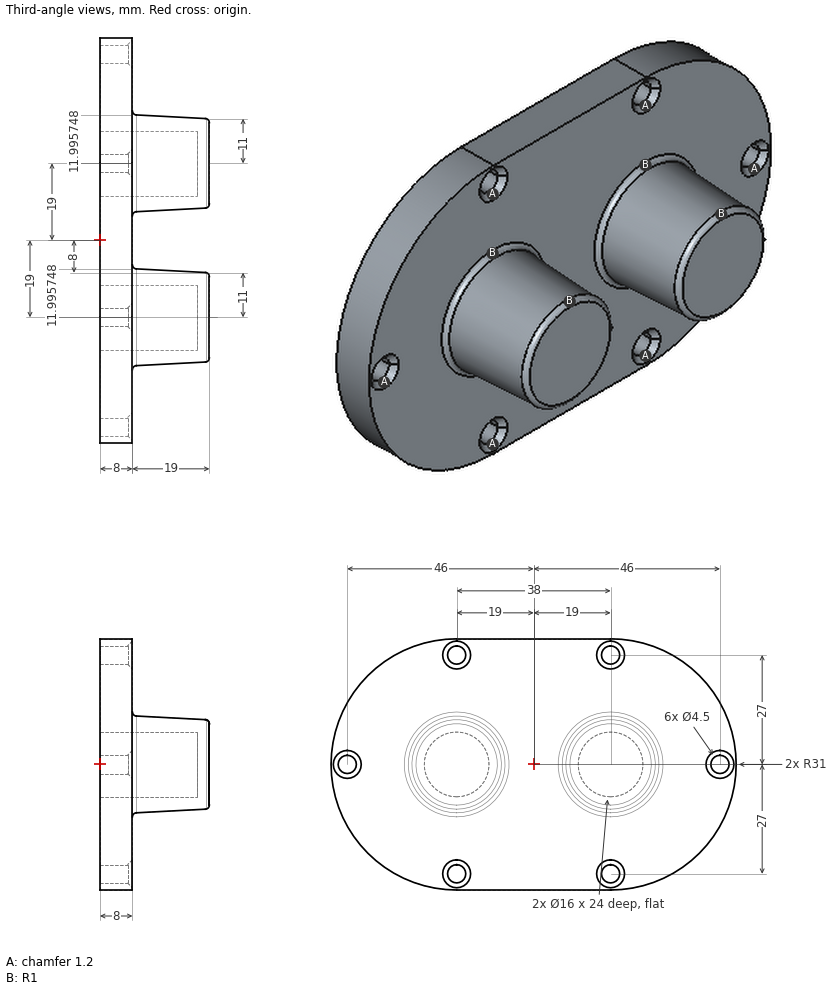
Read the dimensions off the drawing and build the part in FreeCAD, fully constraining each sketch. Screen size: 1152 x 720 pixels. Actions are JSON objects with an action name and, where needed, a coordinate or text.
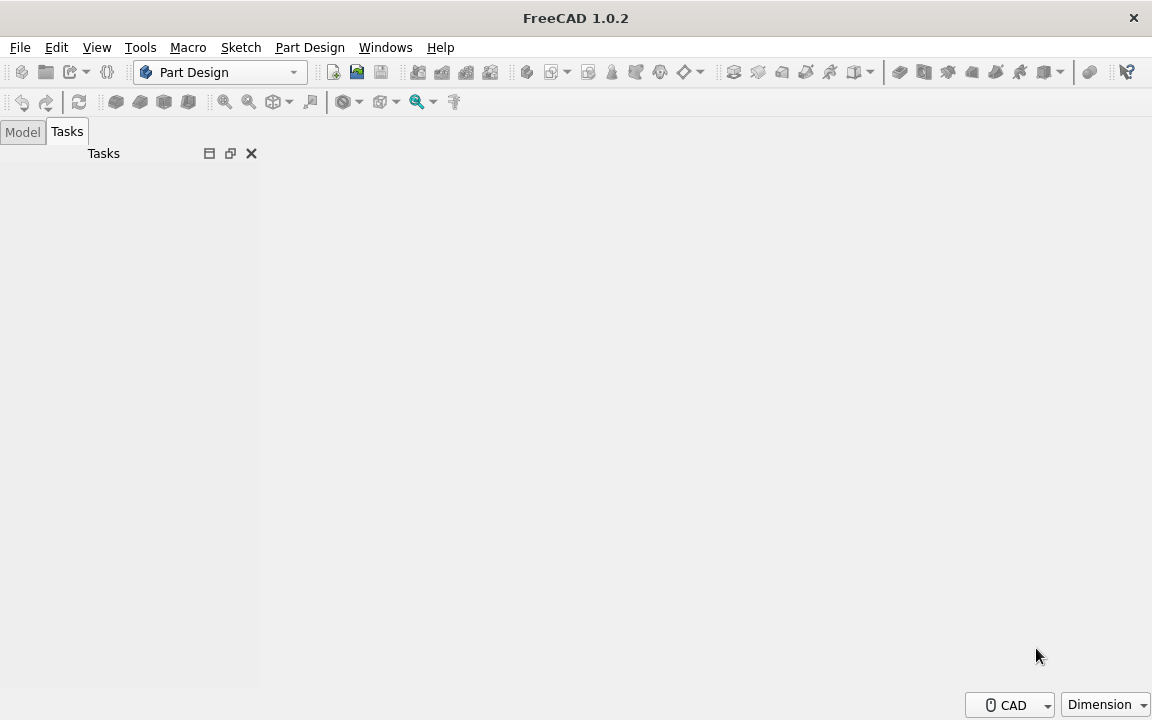
{"action": "left_click", "coordinate": [334, 72]}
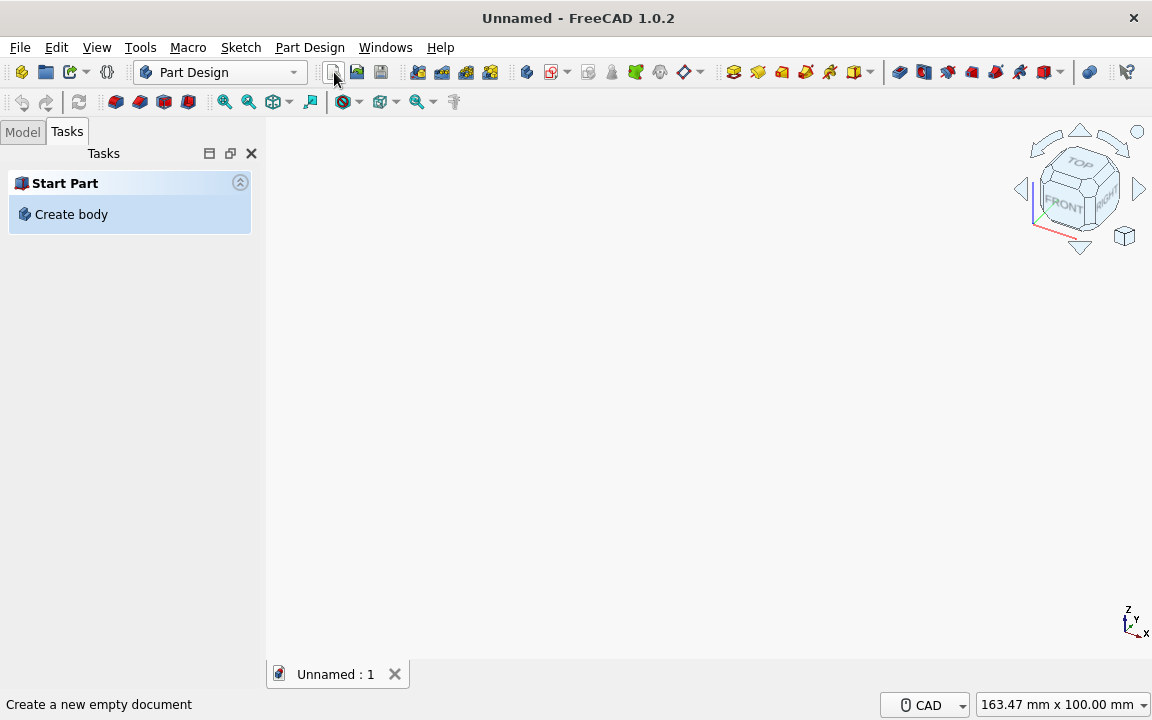
{"action": "left_click", "coordinate": [528, 72]}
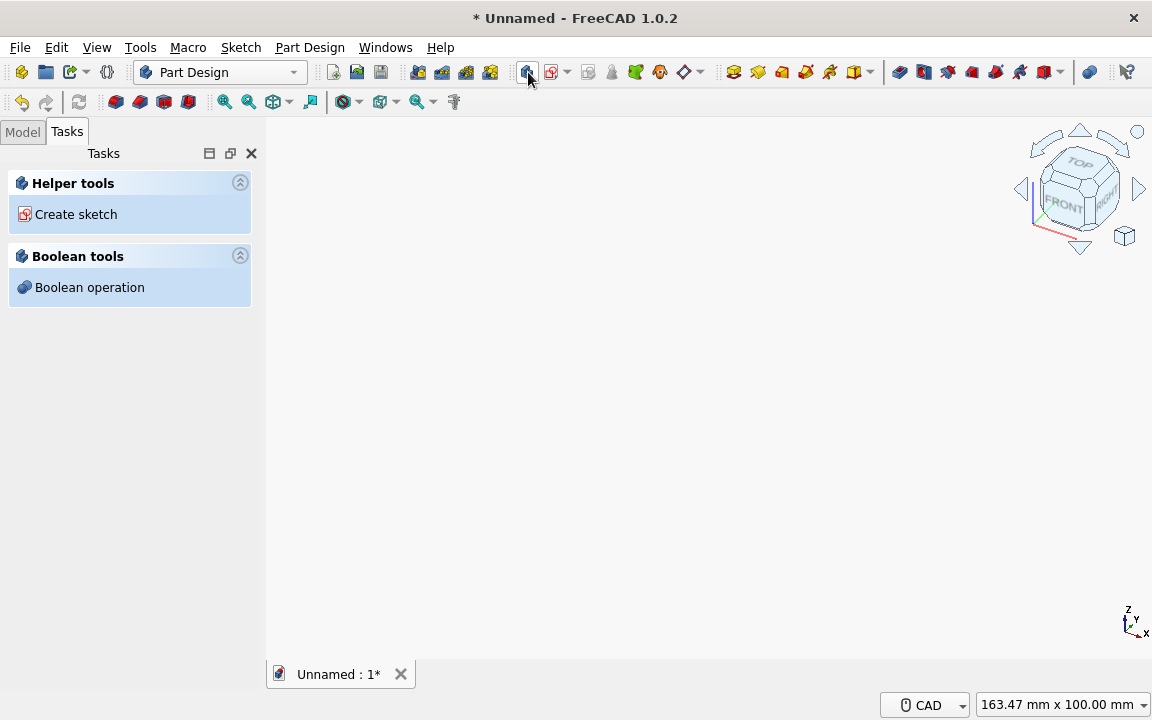
{"action": "left_click", "coordinate": [23, 131]}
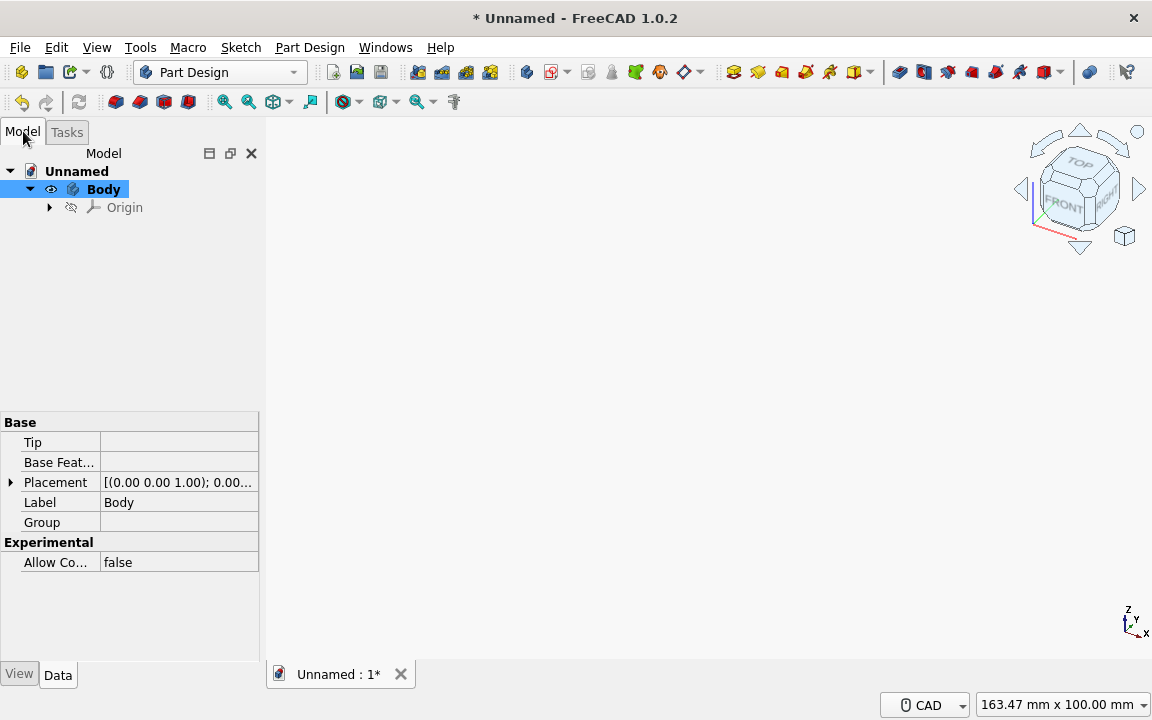
{"action": "left_click", "coordinate": [50, 207]}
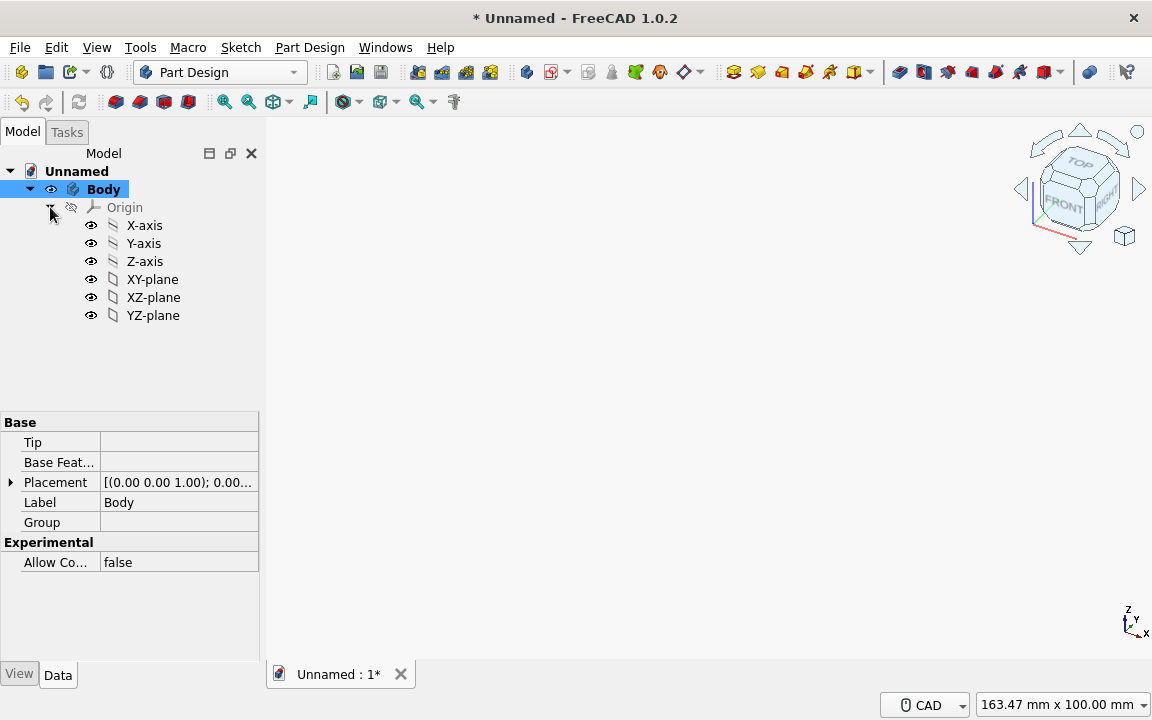
{"action": "left_click", "coordinate": [136, 315]}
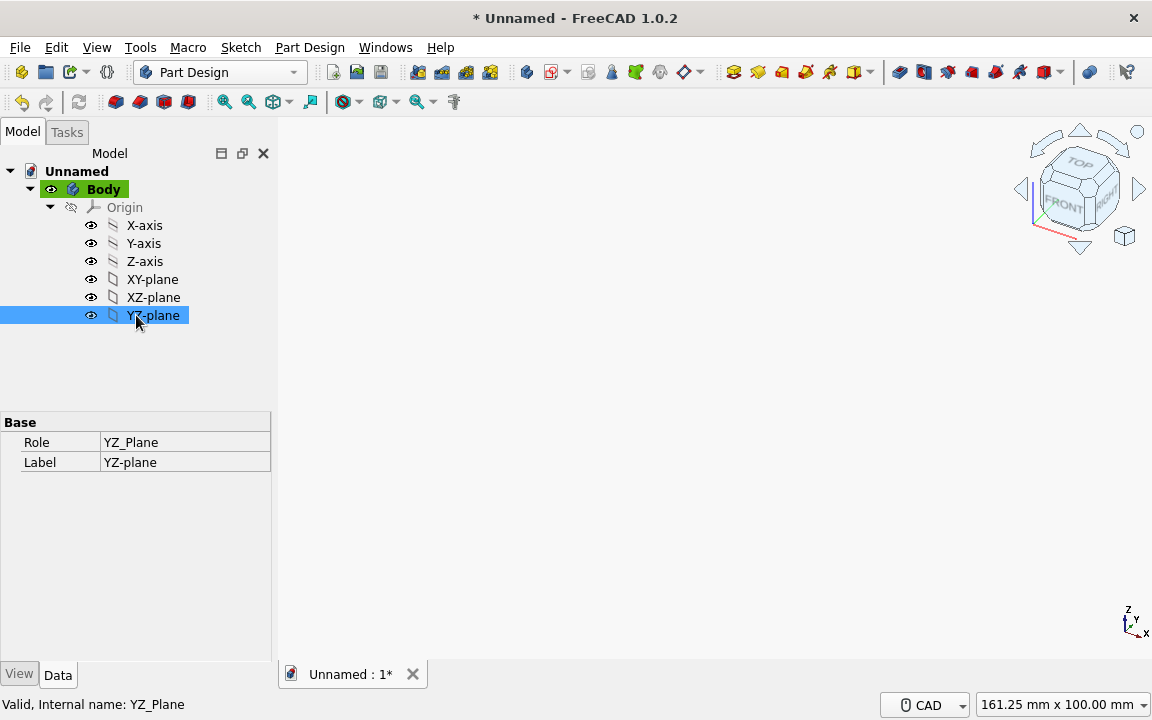
{"action": "left_click", "coordinate": [684, 72]}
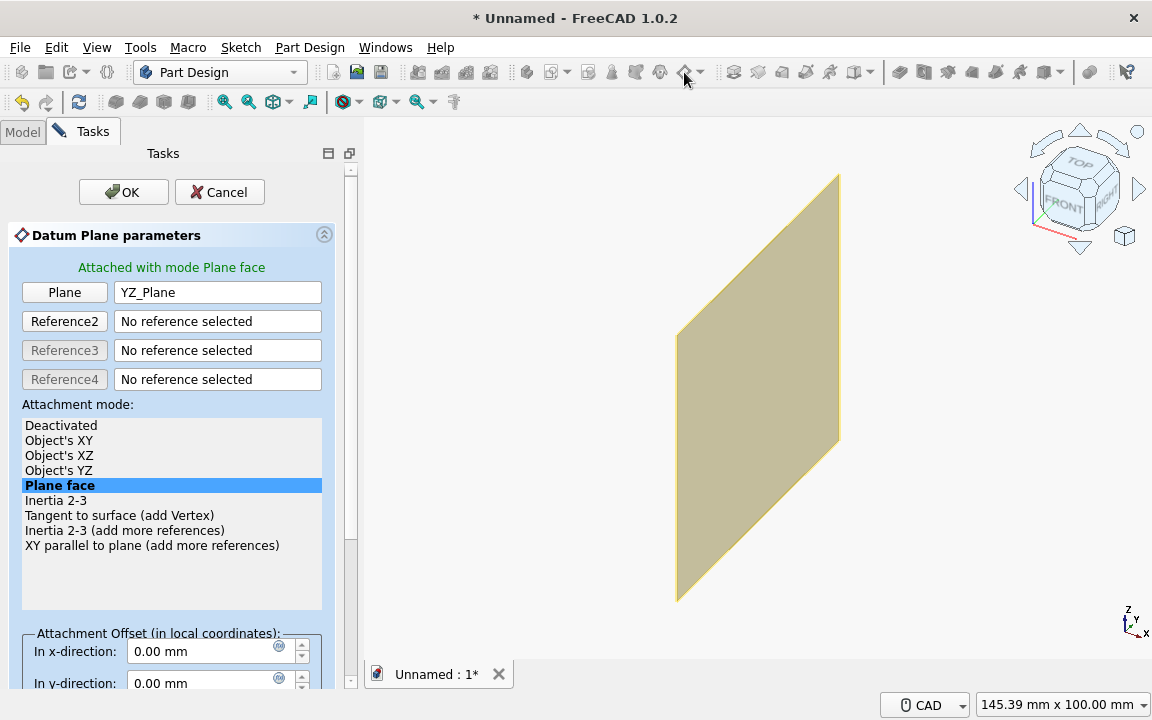
{"action": "scroll", "coordinate": [351, 426], "scroll_direction": "down", "scroll_amount": 2}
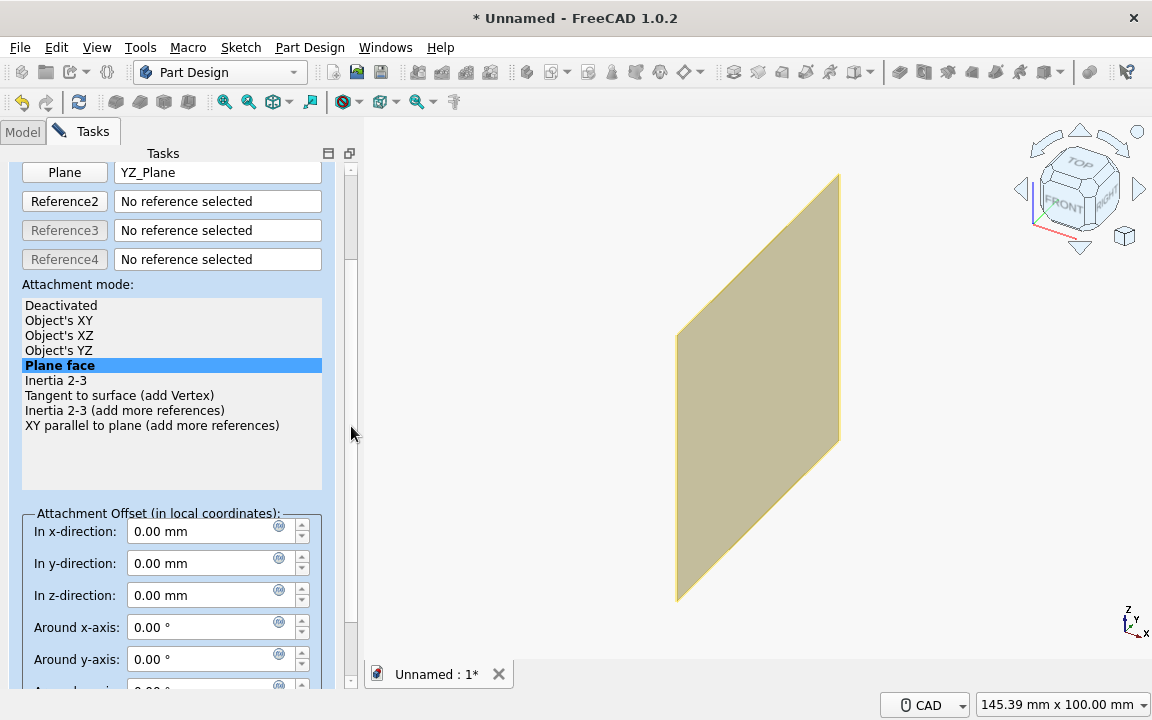
{"action": "triple_click", "coordinate": [210, 595]}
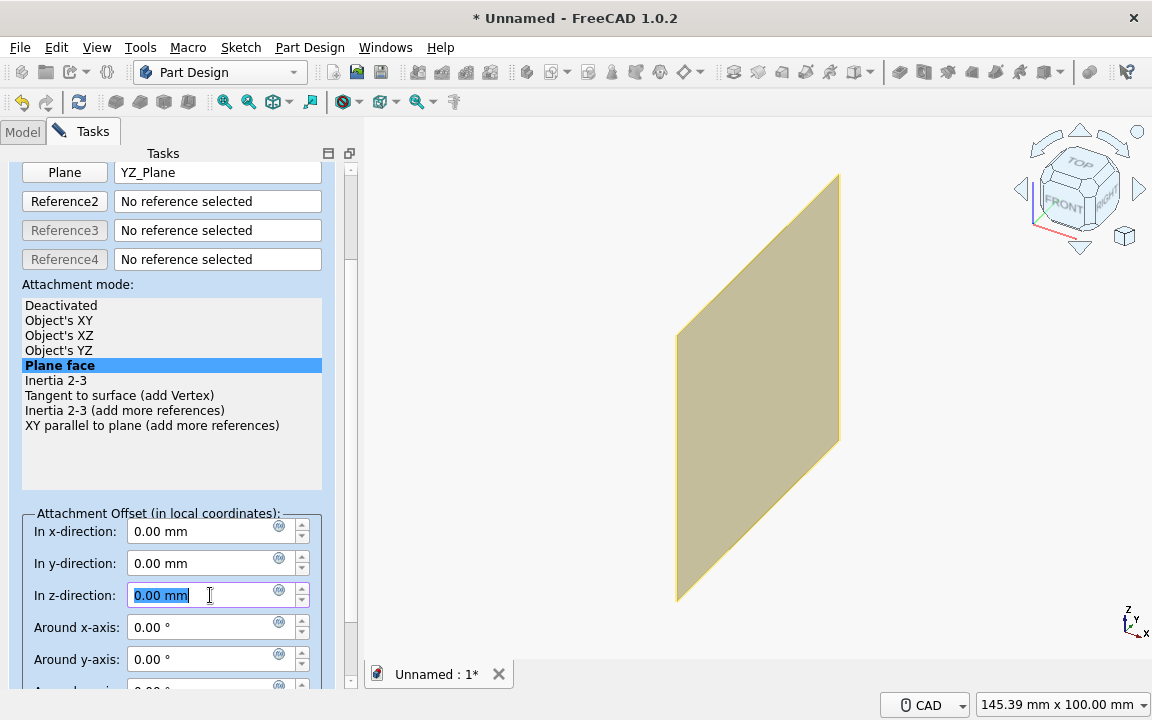
{"action": "type", "text": "8"}
{"action": "key", "text": "Tab"}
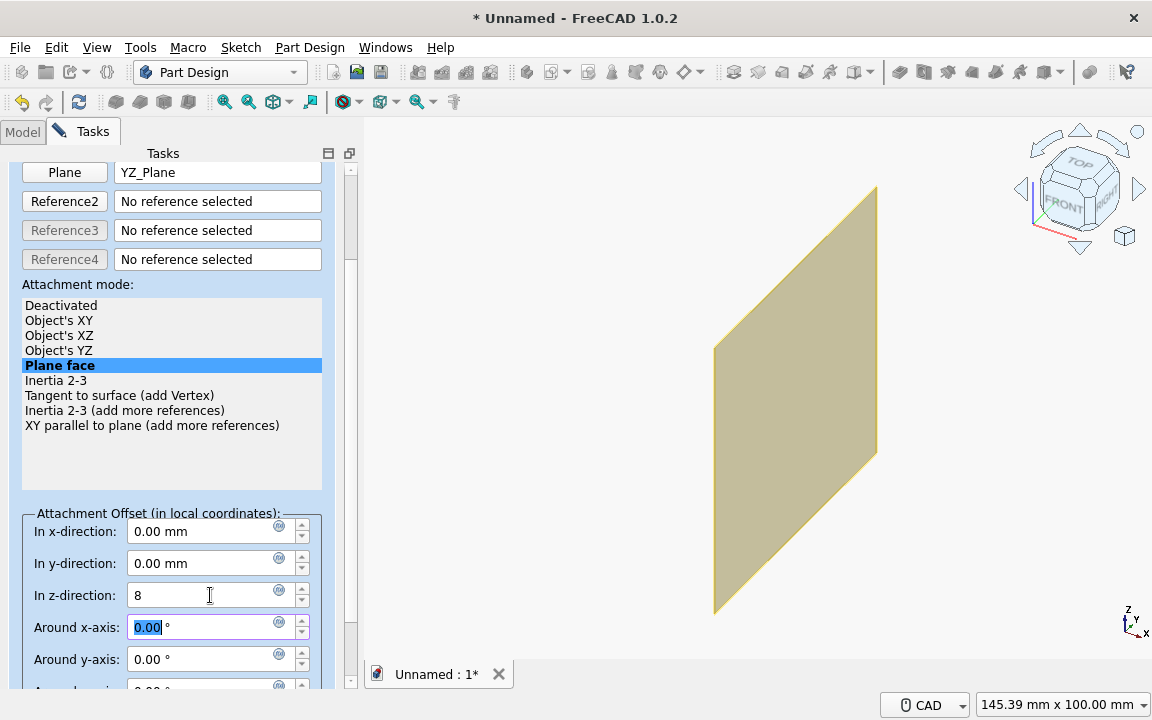
{"action": "scroll", "coordinate": [351, 426], "scroll_direction": "up", "scroll_amount": 3}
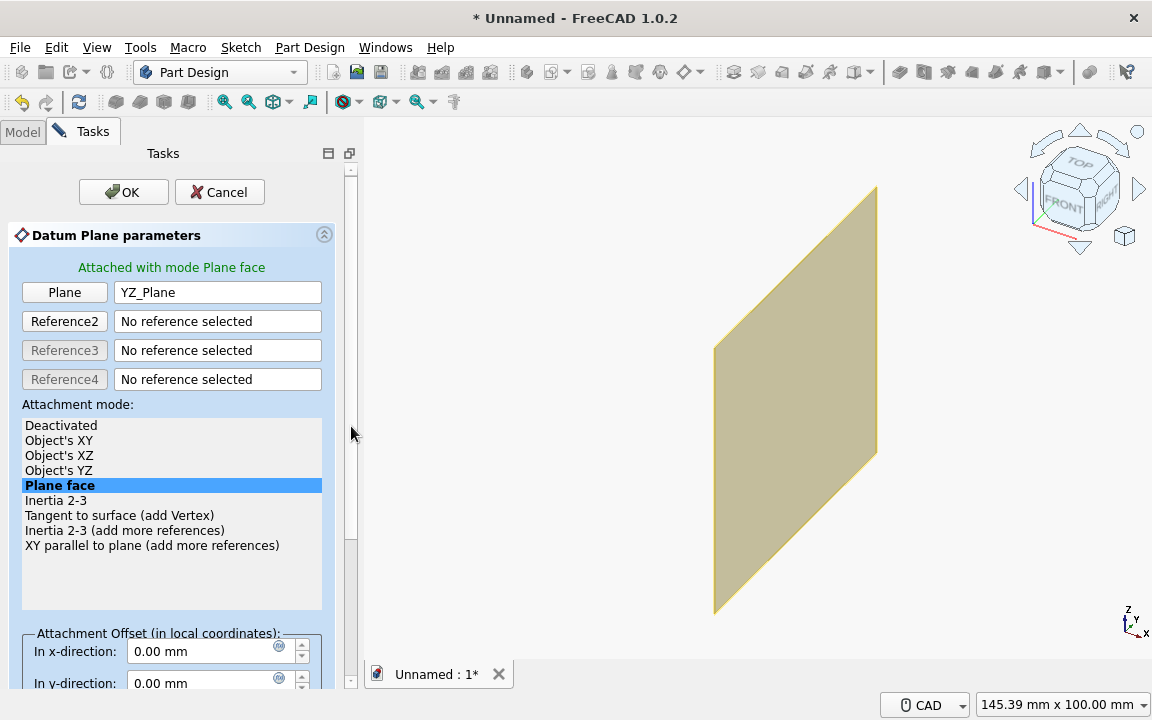
{"action": "left_click", "coordinate": [124, 192]}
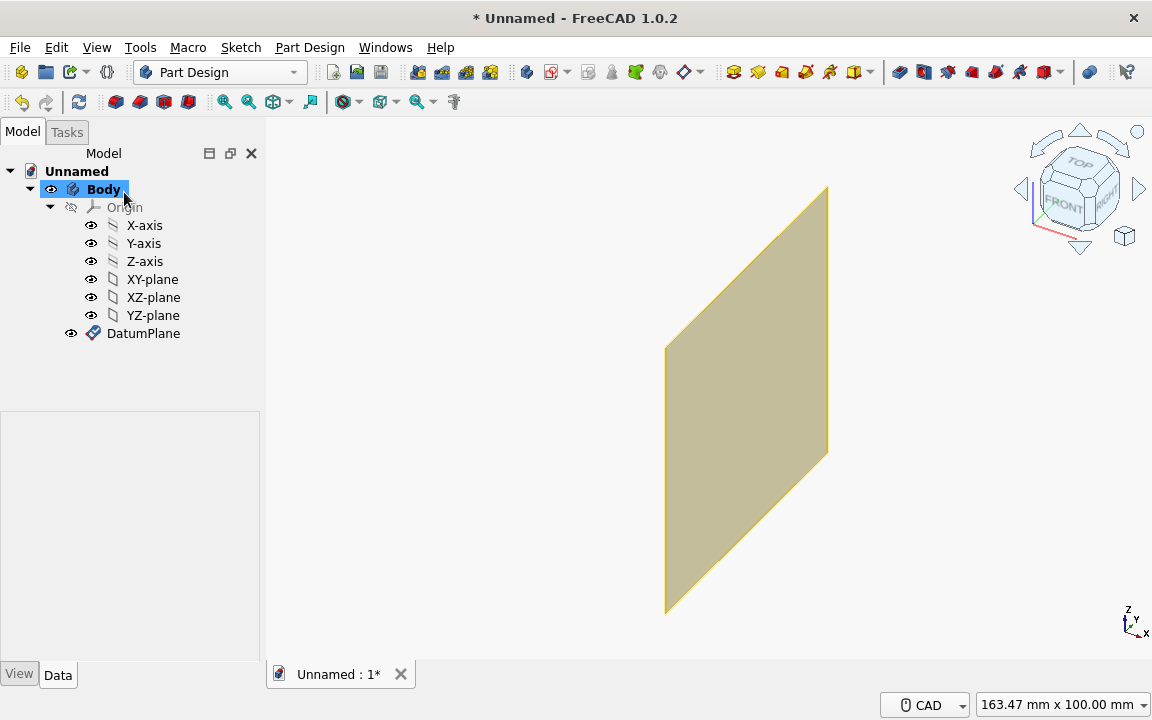
{"action": "left_click", "coordinate": [116, 333]}